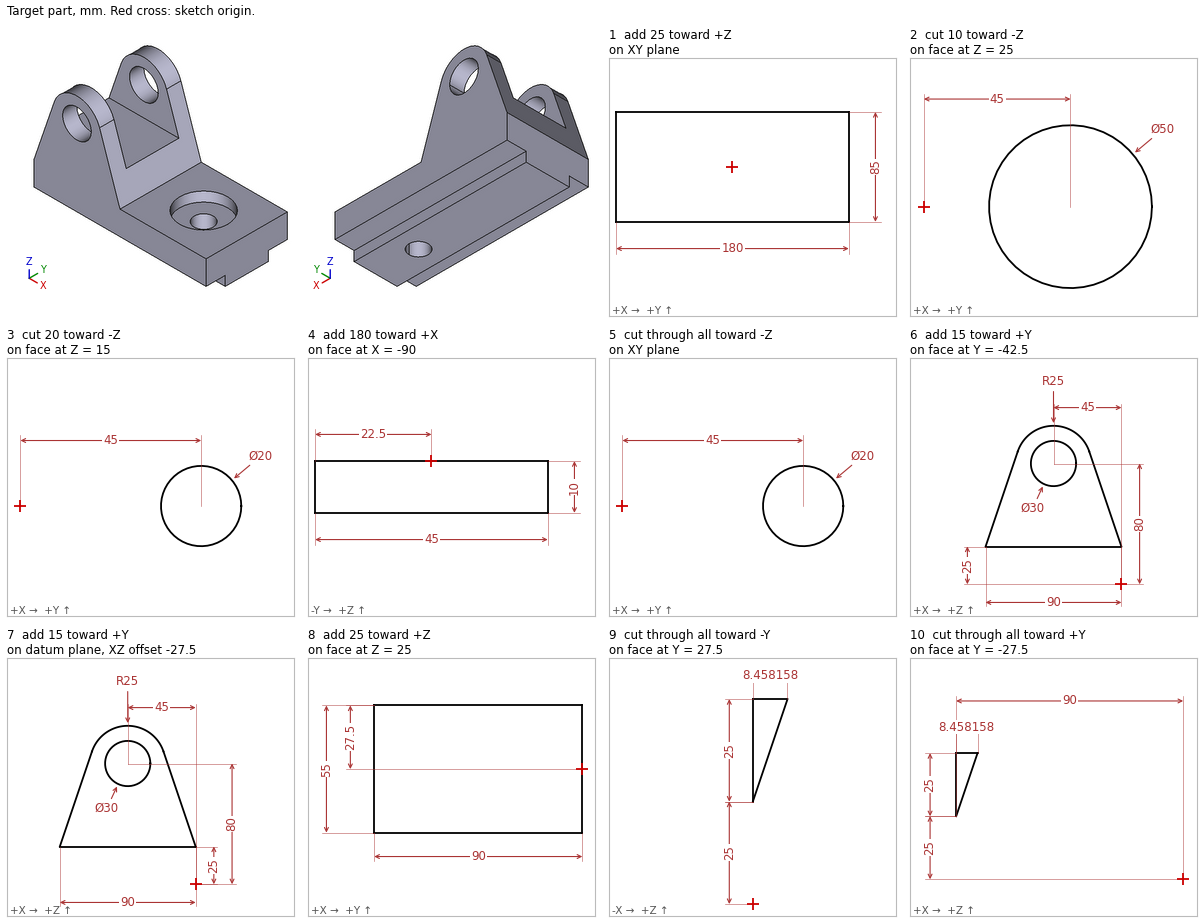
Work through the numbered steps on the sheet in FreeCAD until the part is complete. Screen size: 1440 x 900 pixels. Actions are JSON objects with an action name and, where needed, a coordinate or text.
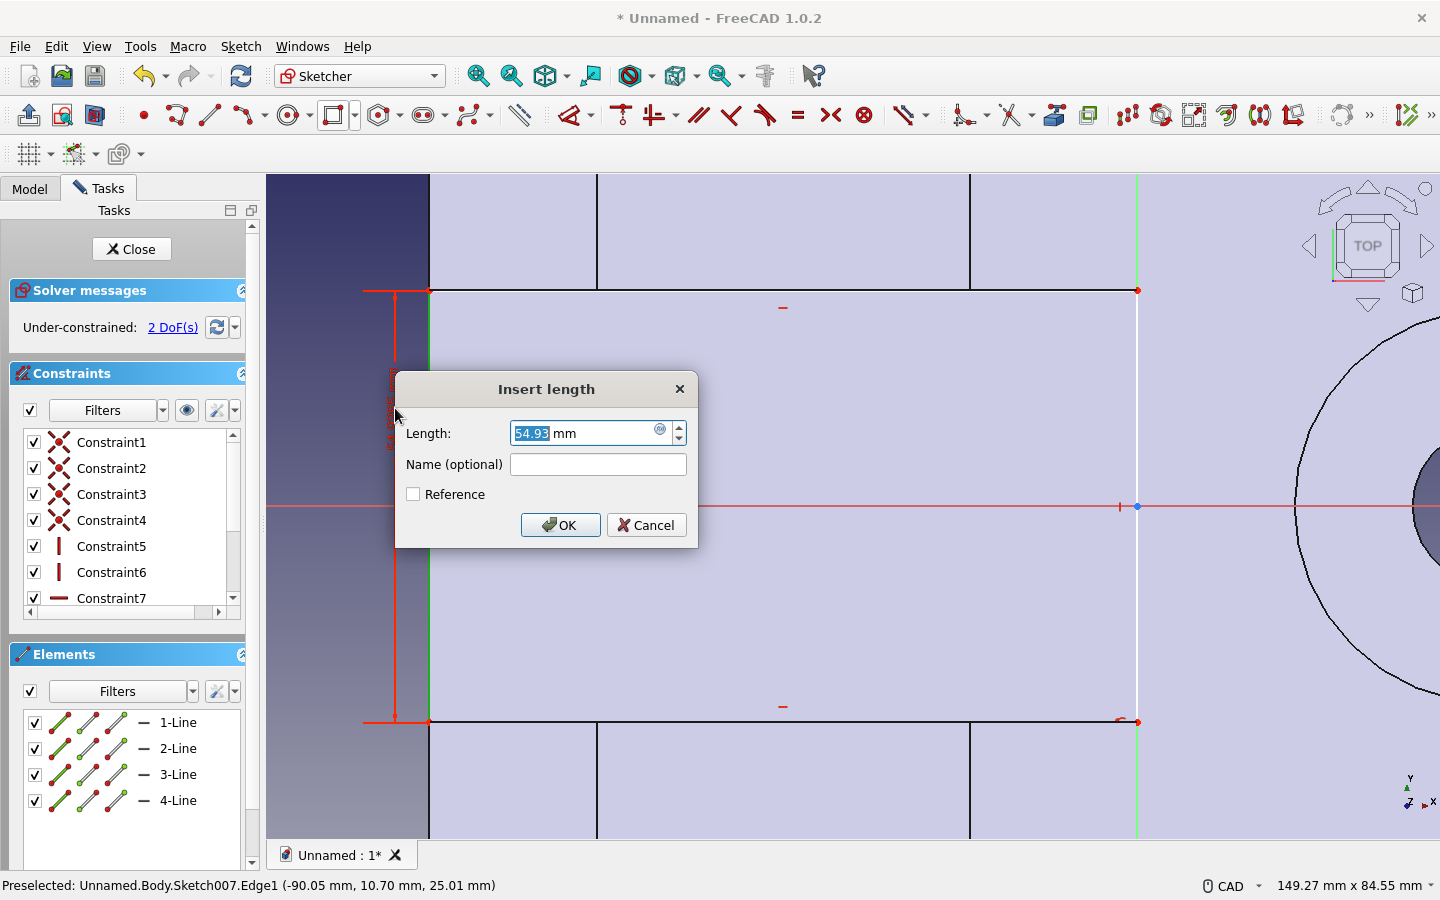
{"action": "type", "text": "55"}
{"action": "key", "text": "Return"}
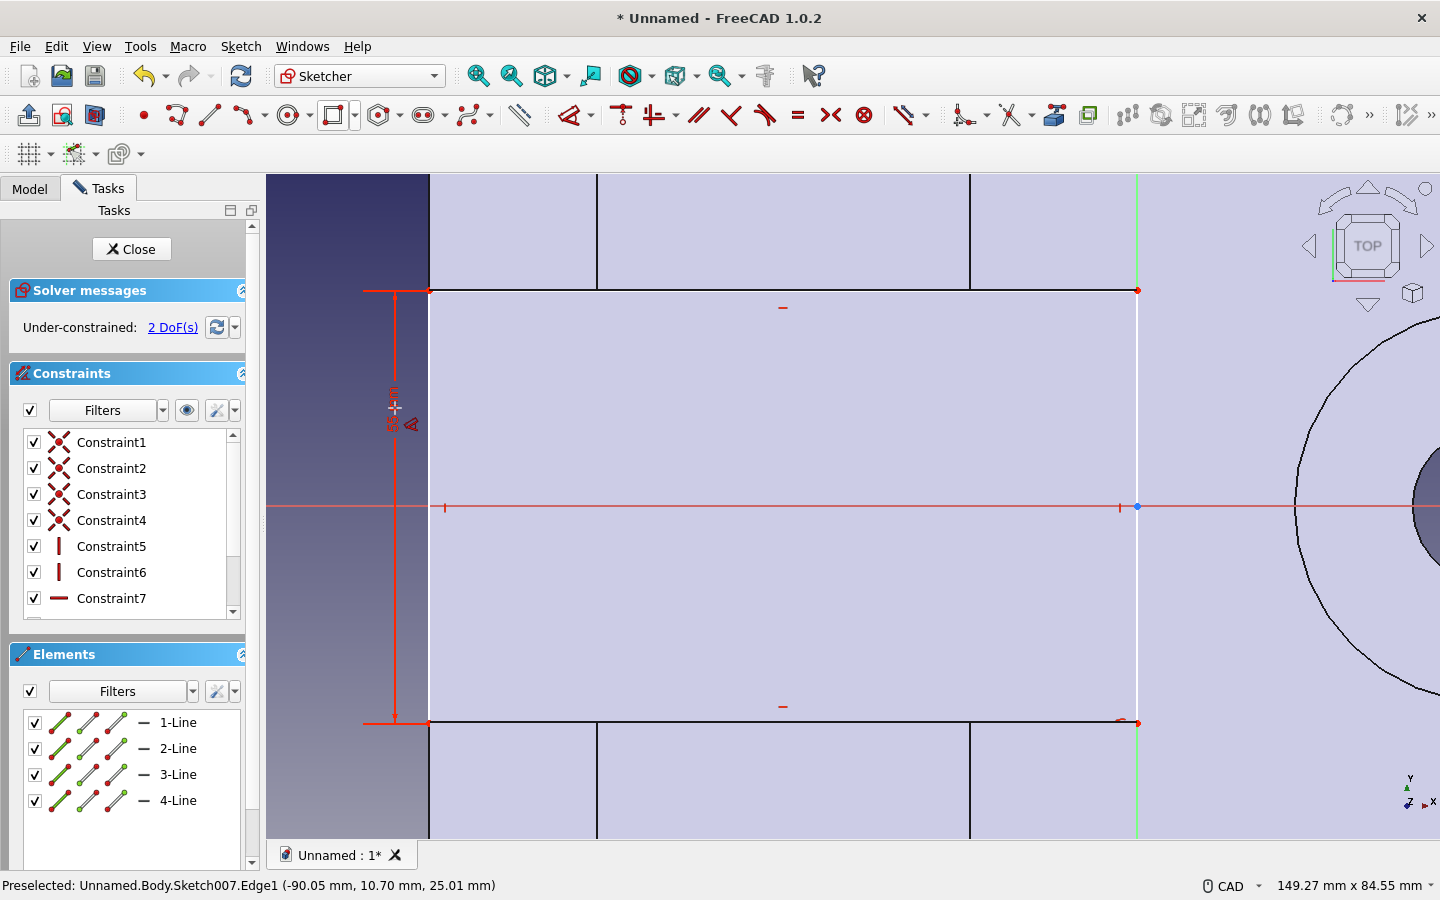
{"action": "left_click", "coordinate": [641, 724]}
{"action": "left_click", "coordinate": [783, 758]}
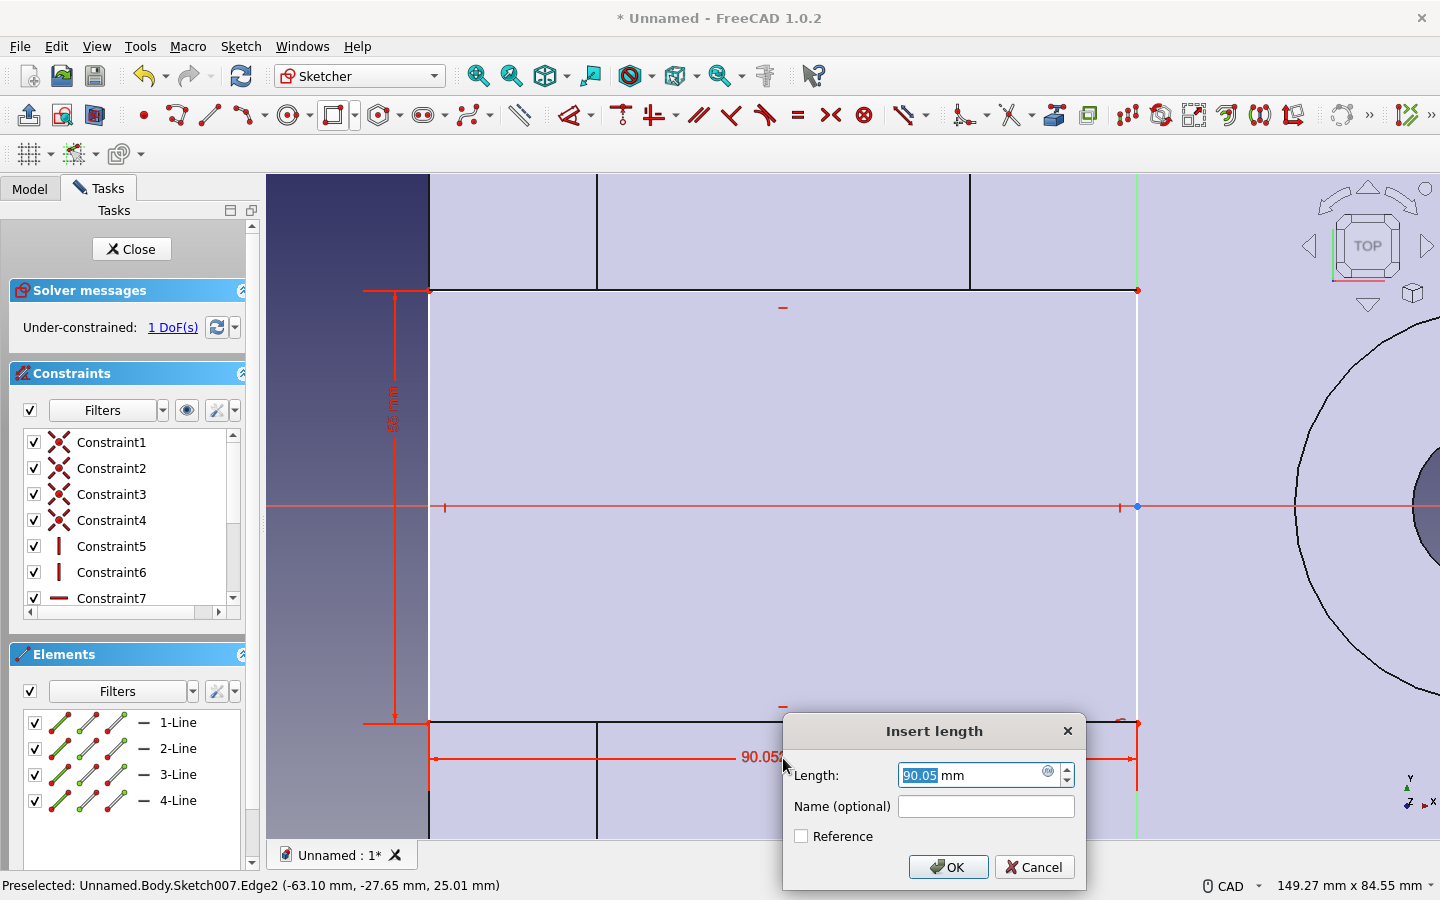
{"action": "type", "text": "90"}
{"action": "key", "text": "Return"}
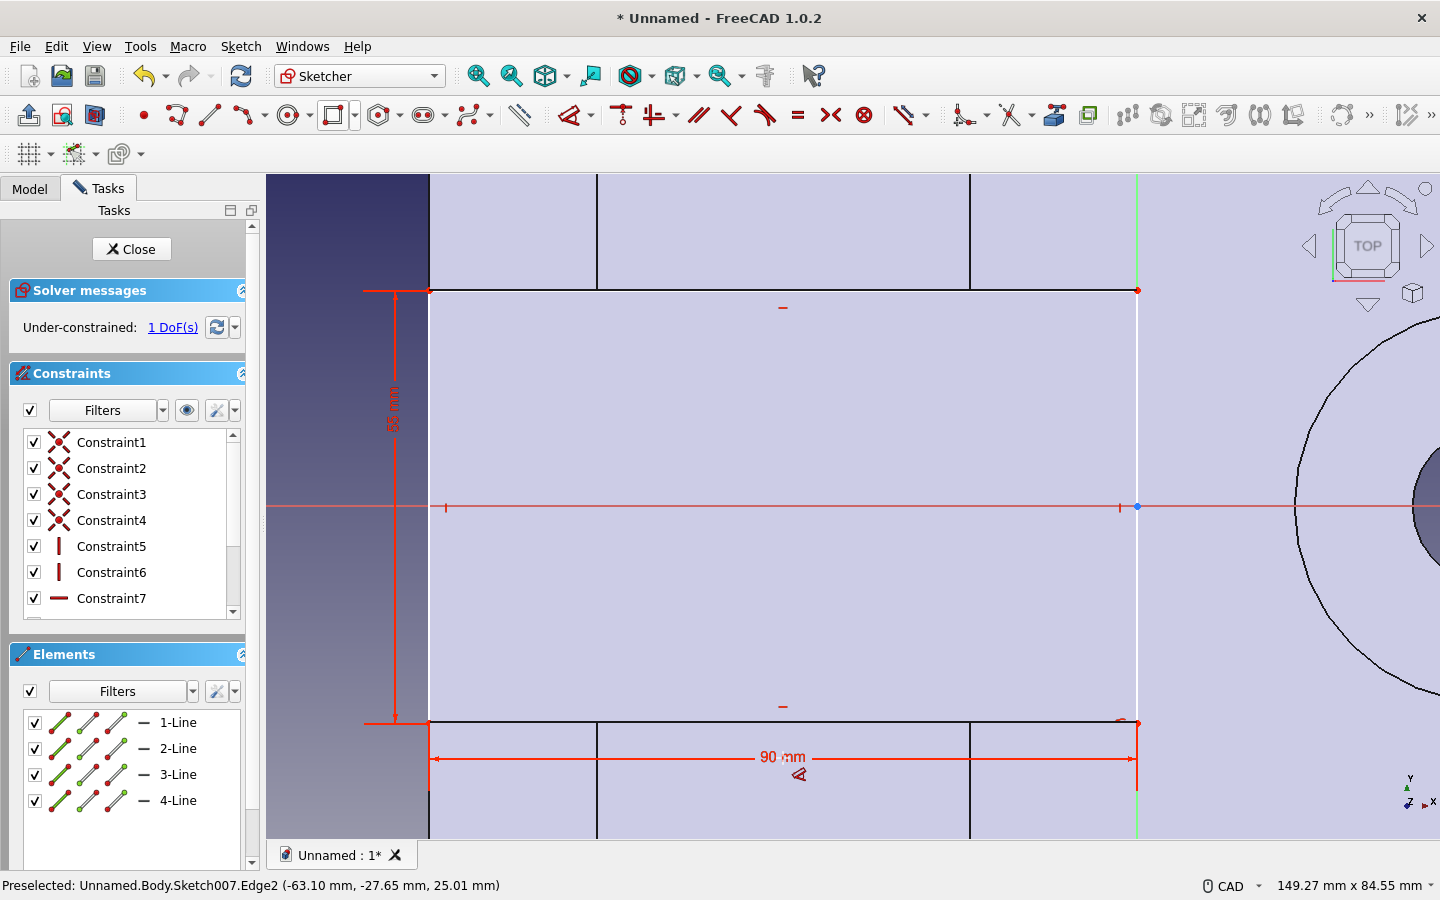
{"action": "left_click", "coordinate": [429, 291]}
{"action": "left_click", "coordinate": [1171, 399]}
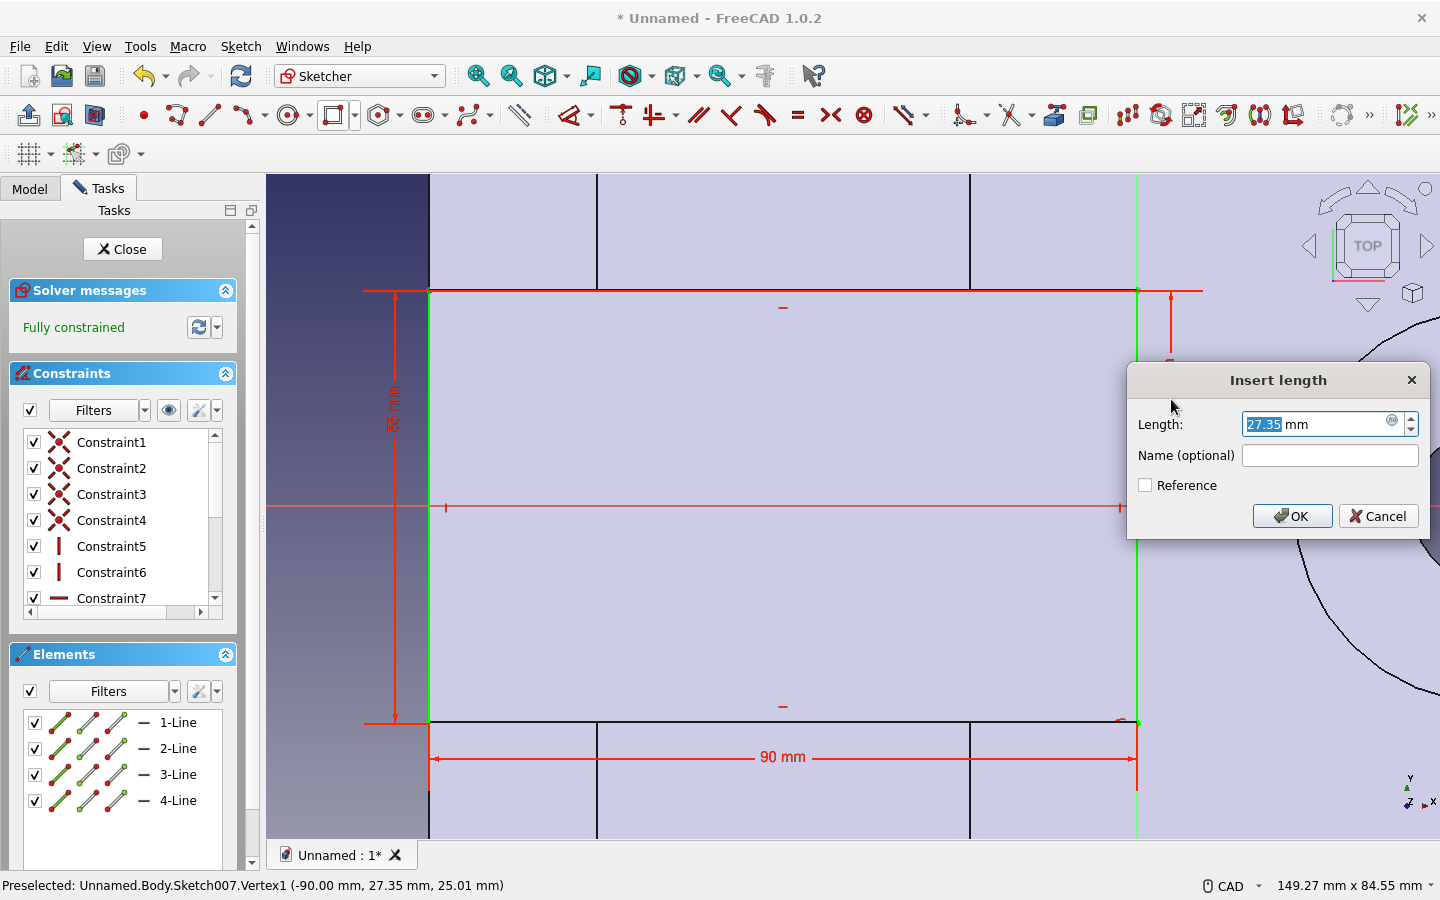
{"action": "type", "text": "27.5"}
{"action": "key", "text": "Return"}
{"action": "key", "text": "Escape"}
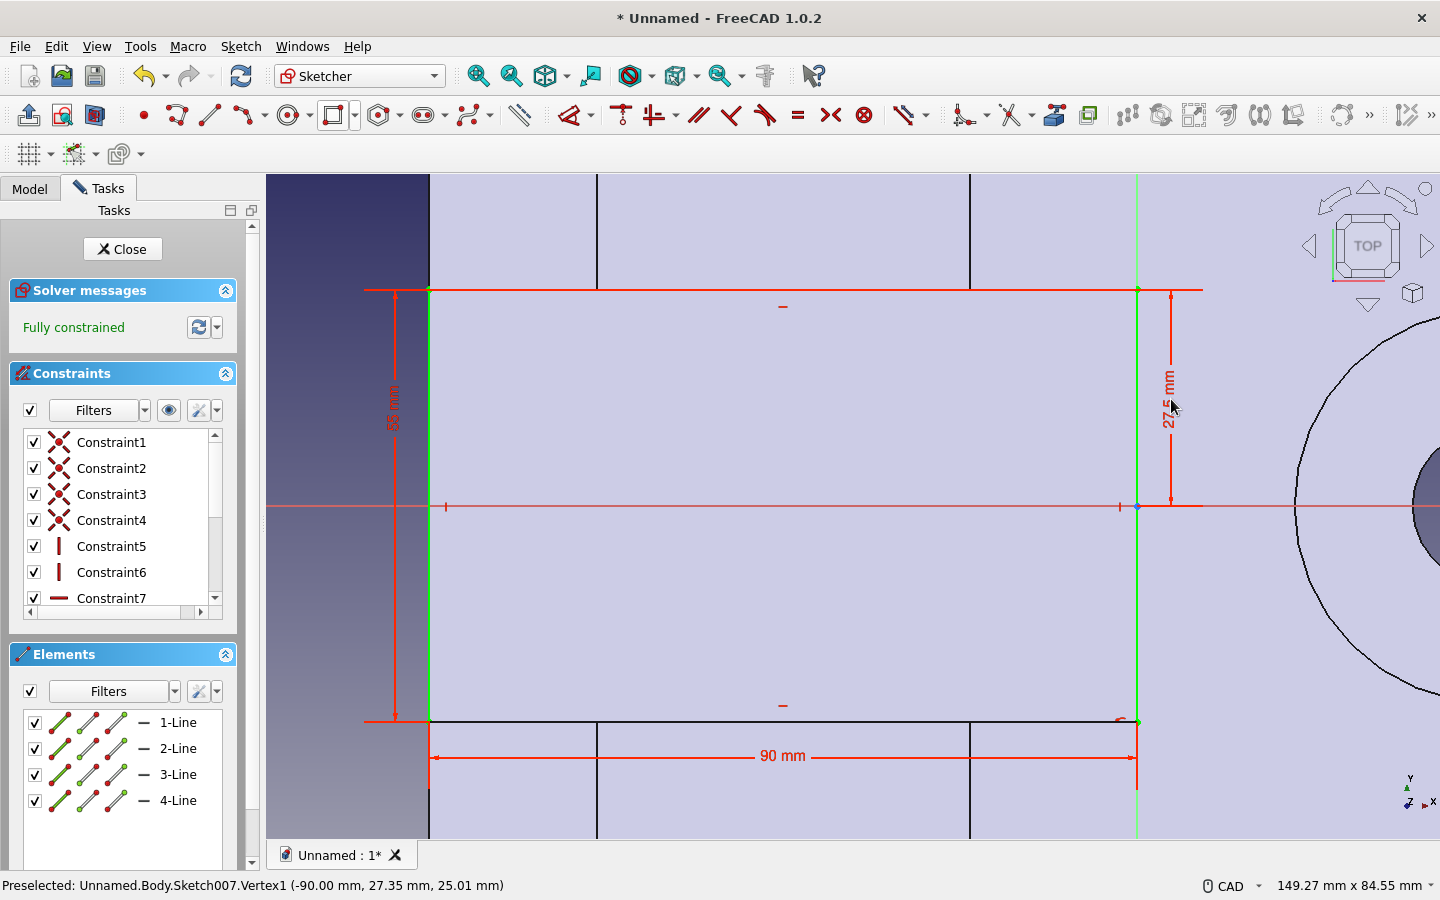
{"action": "left_click", "coordinate": [123, 249]}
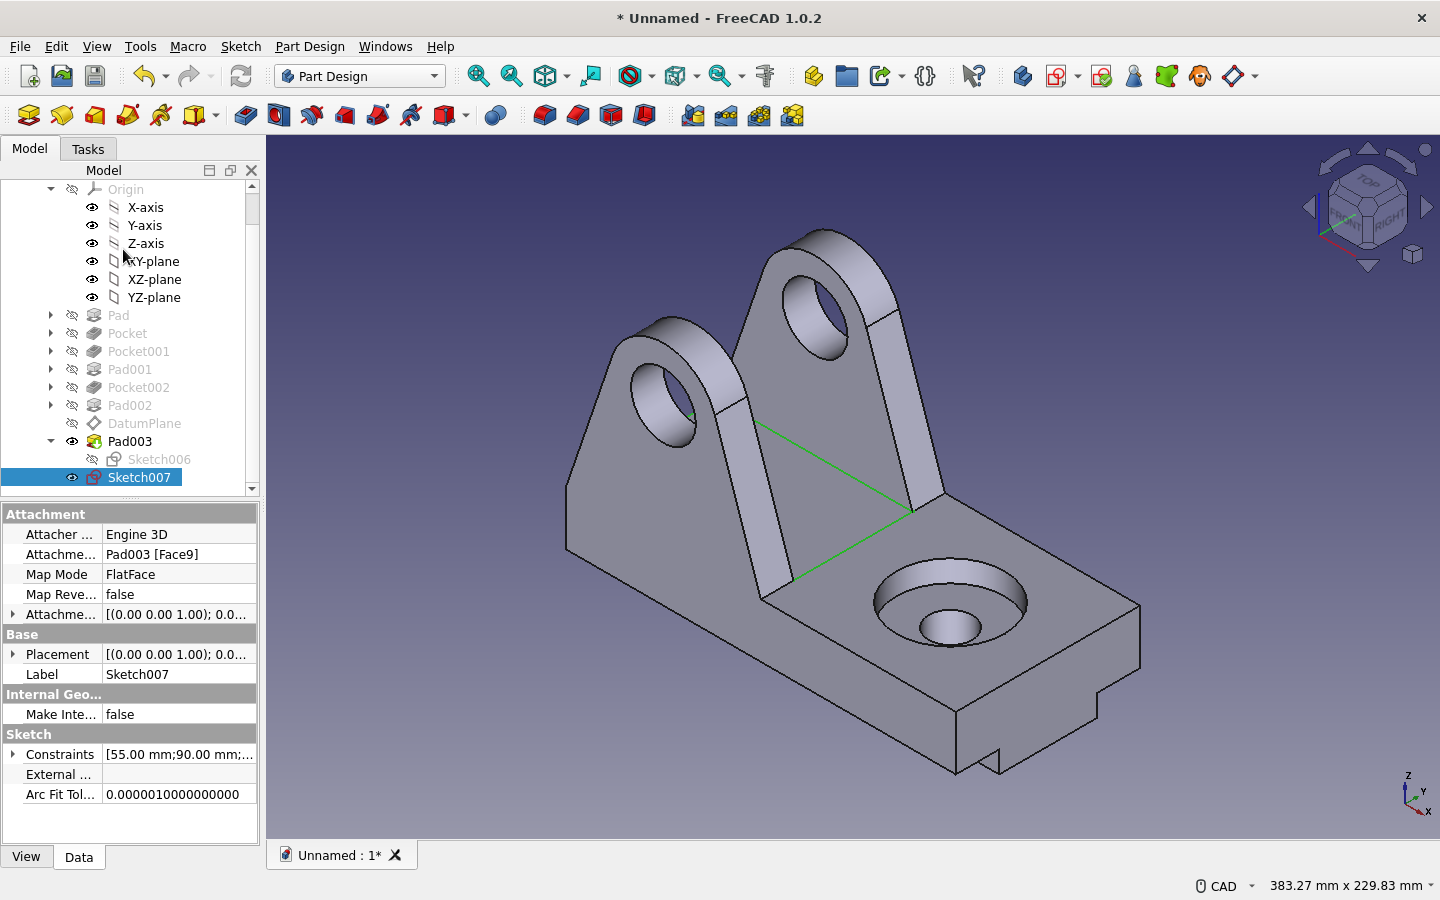
{"action": "left_click", "coordinate": [29, 116]}